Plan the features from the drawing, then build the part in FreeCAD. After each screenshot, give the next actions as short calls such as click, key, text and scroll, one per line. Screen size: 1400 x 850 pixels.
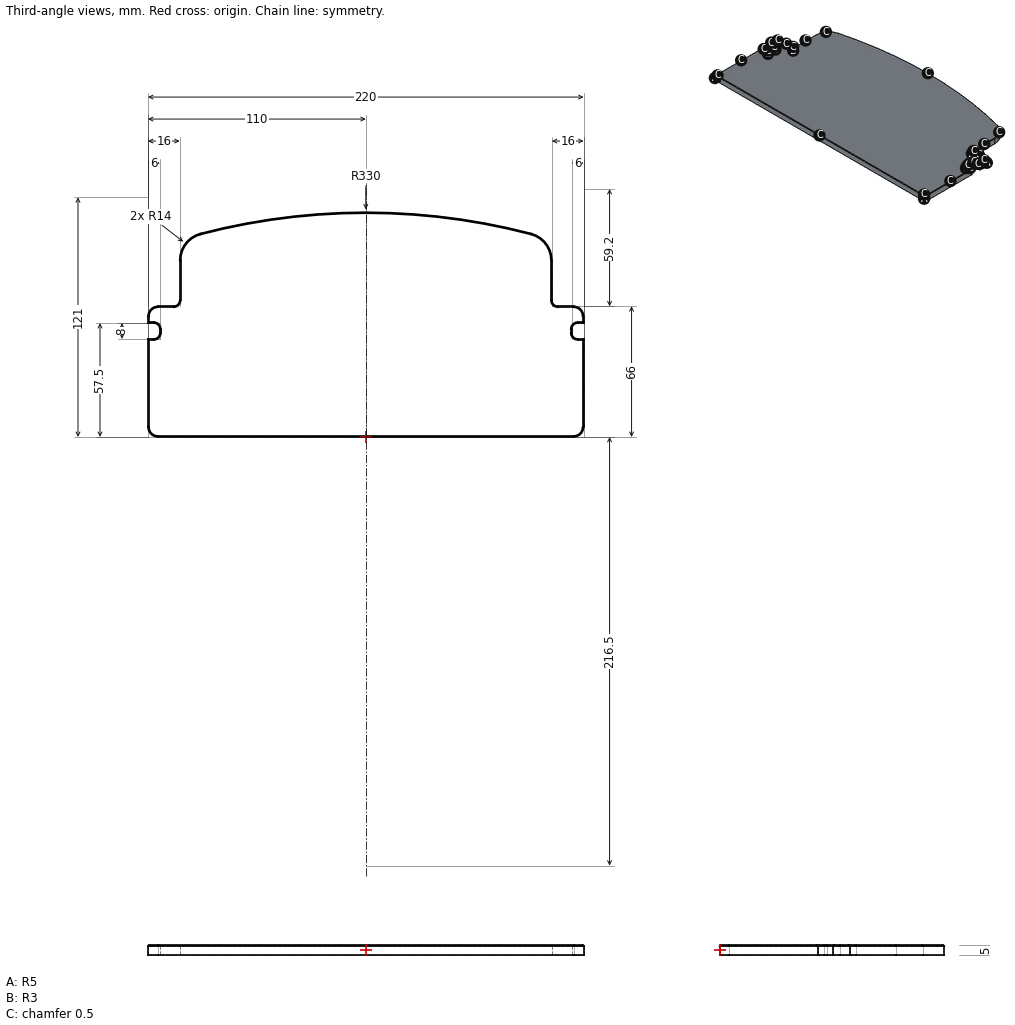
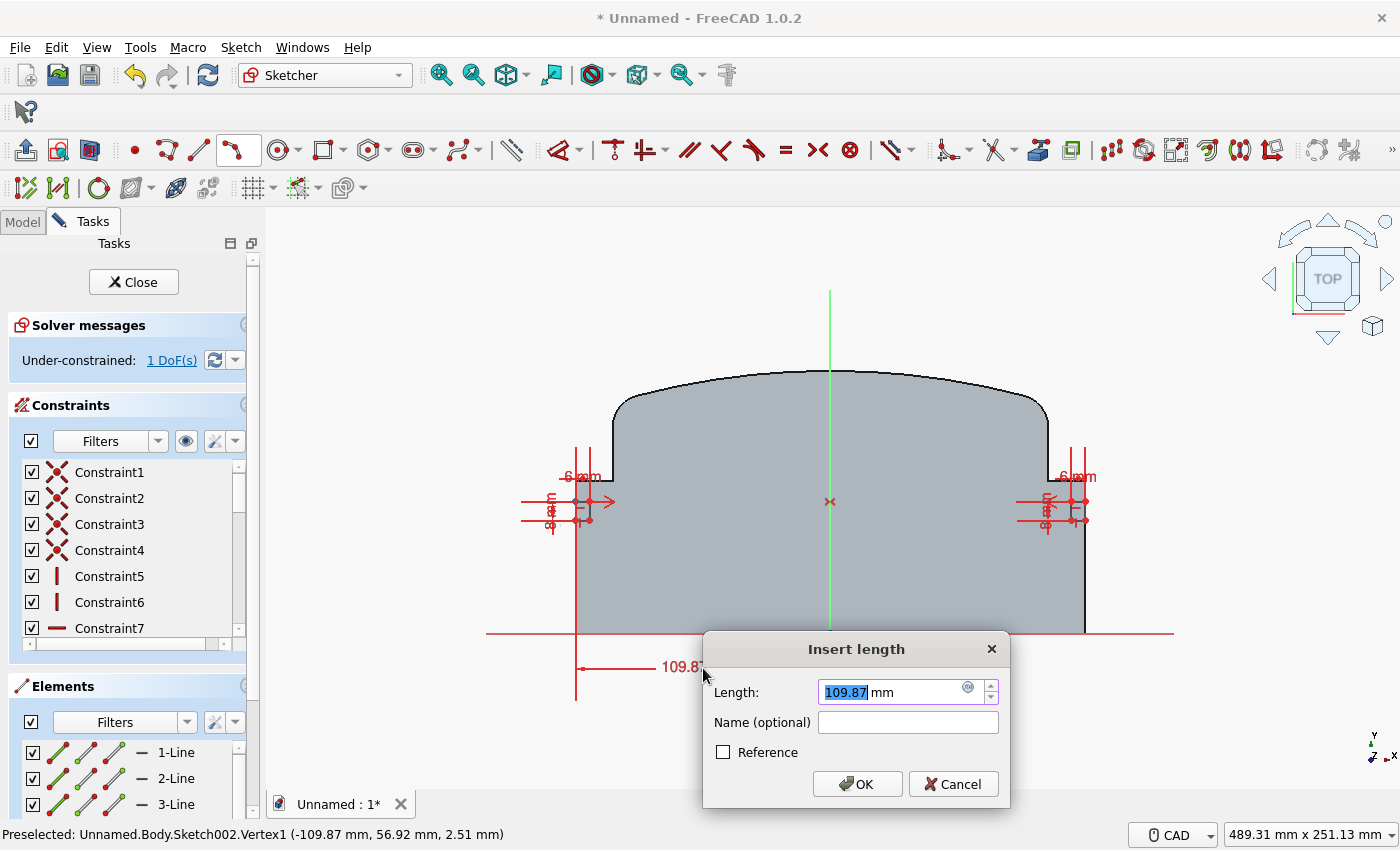
text(110)
key(Return)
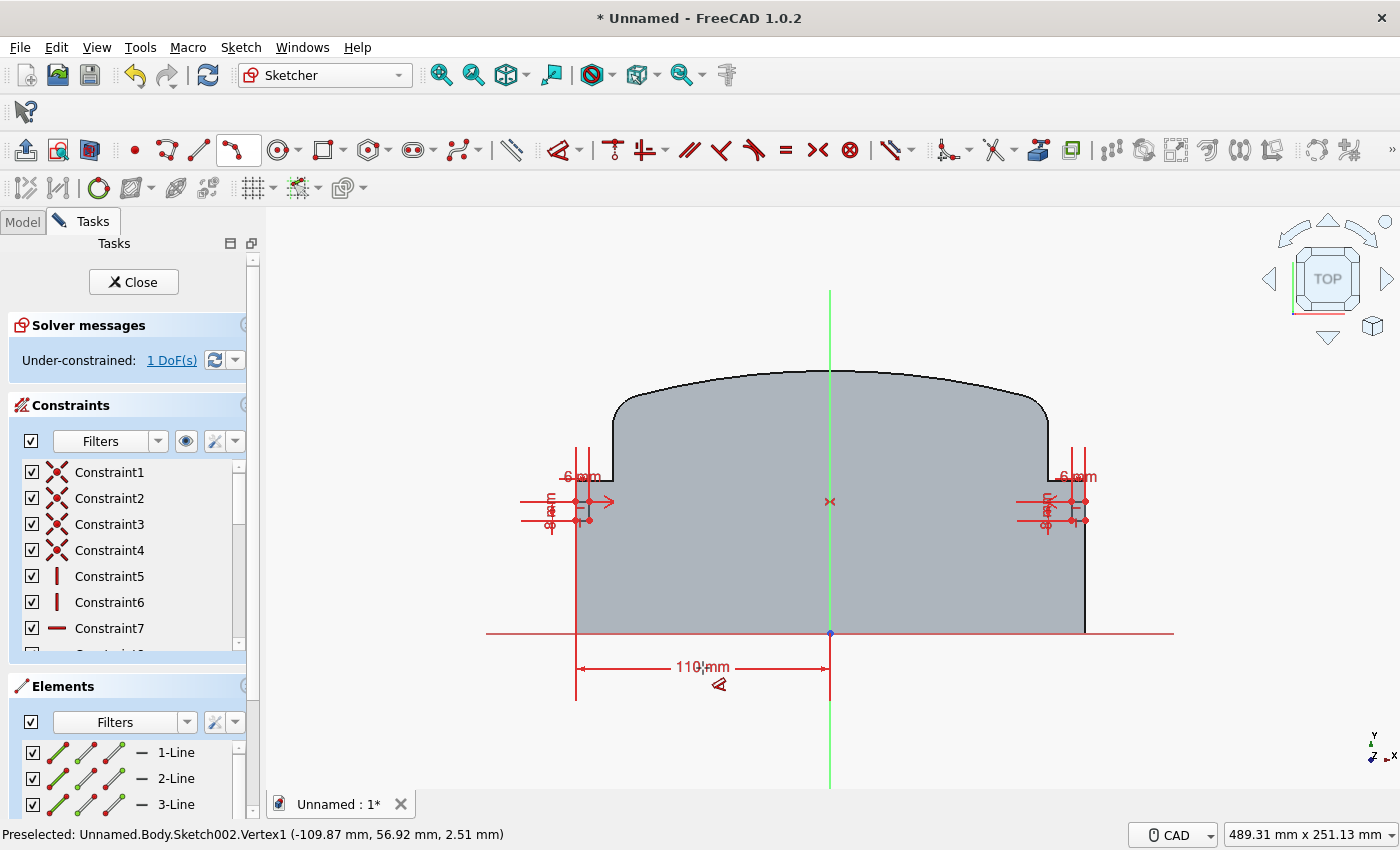
click(576, 502)
click(542, 568)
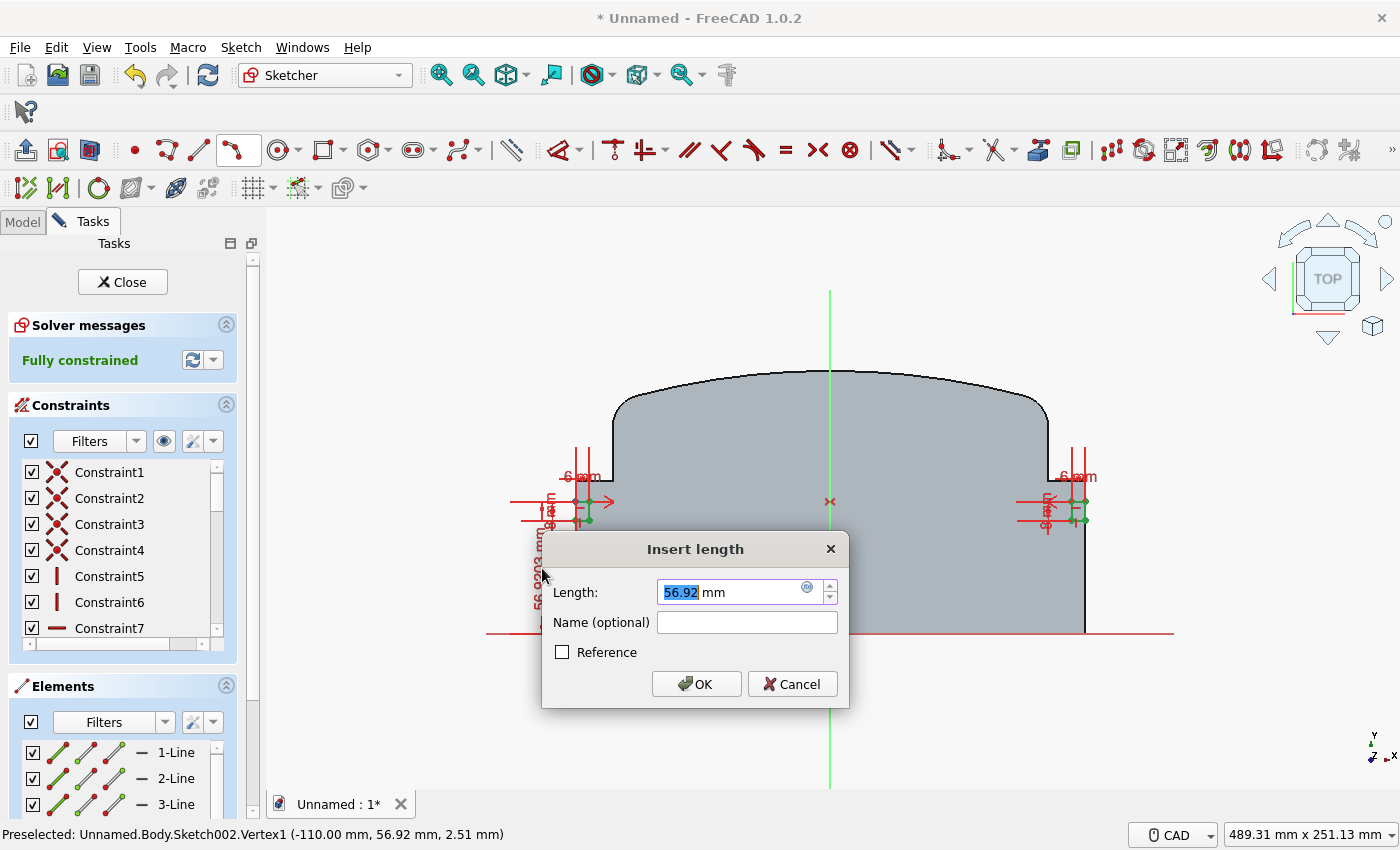
text(57.5)
key(Return)
key(Escape)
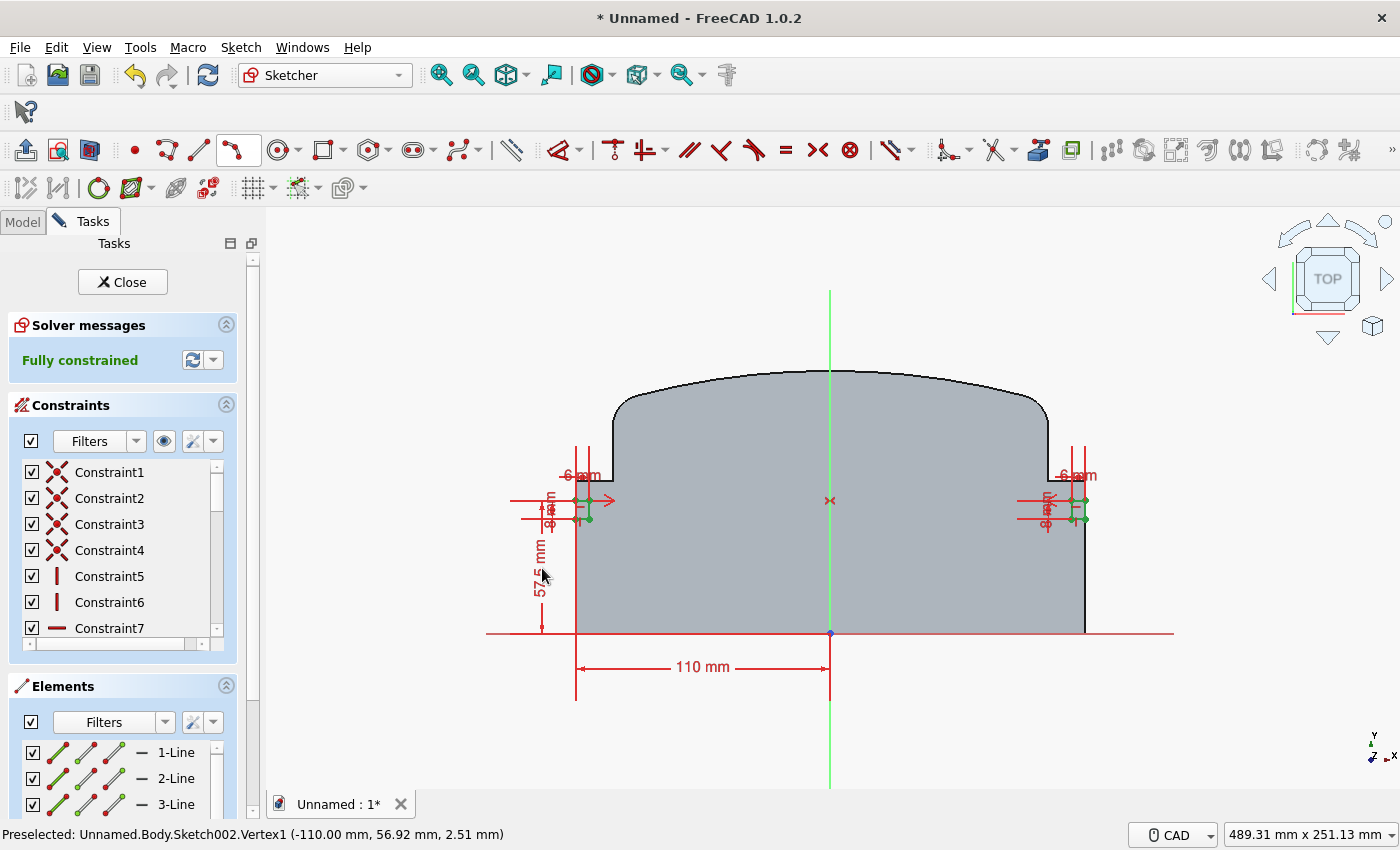
click(123, 282)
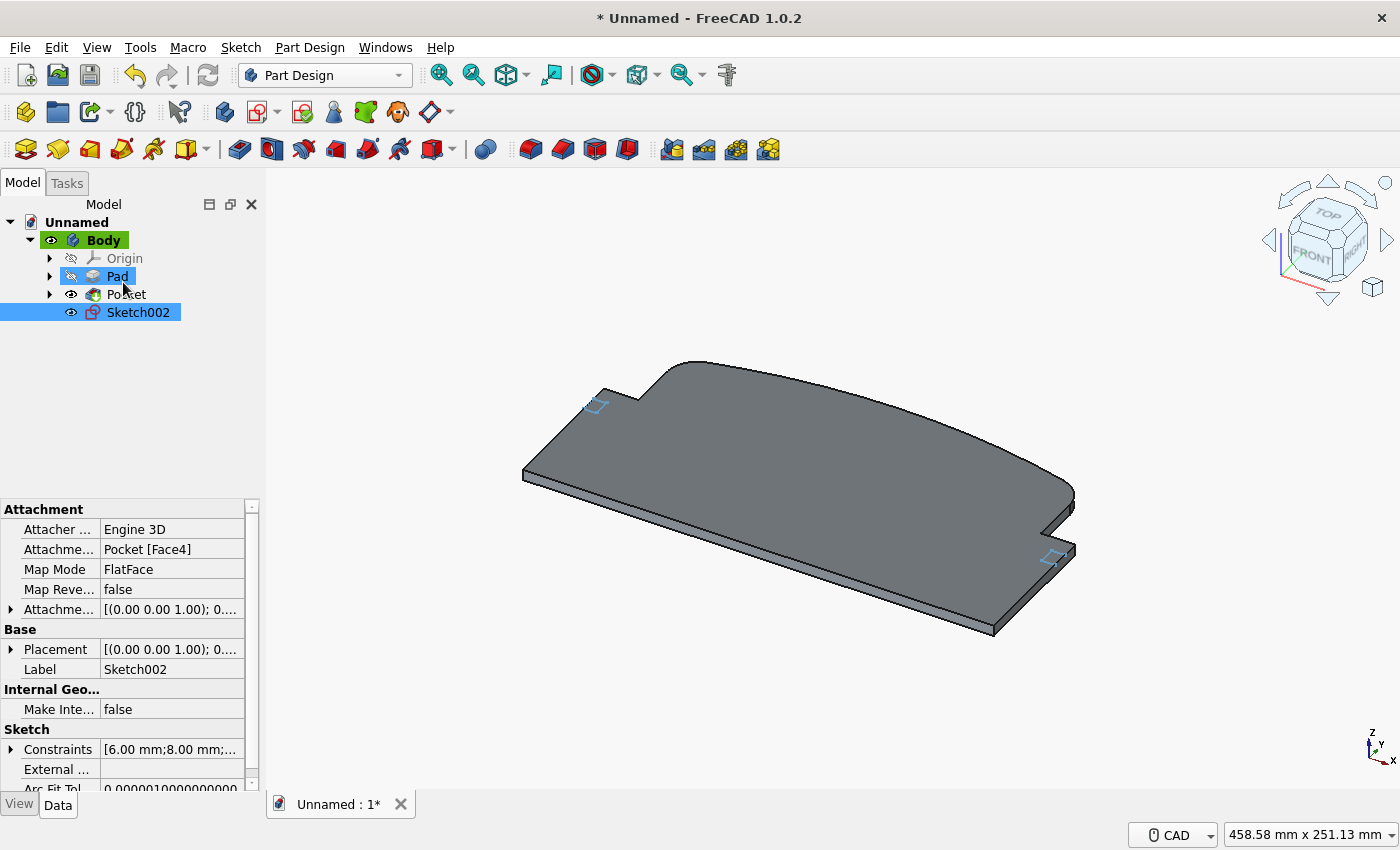
click(240, 150)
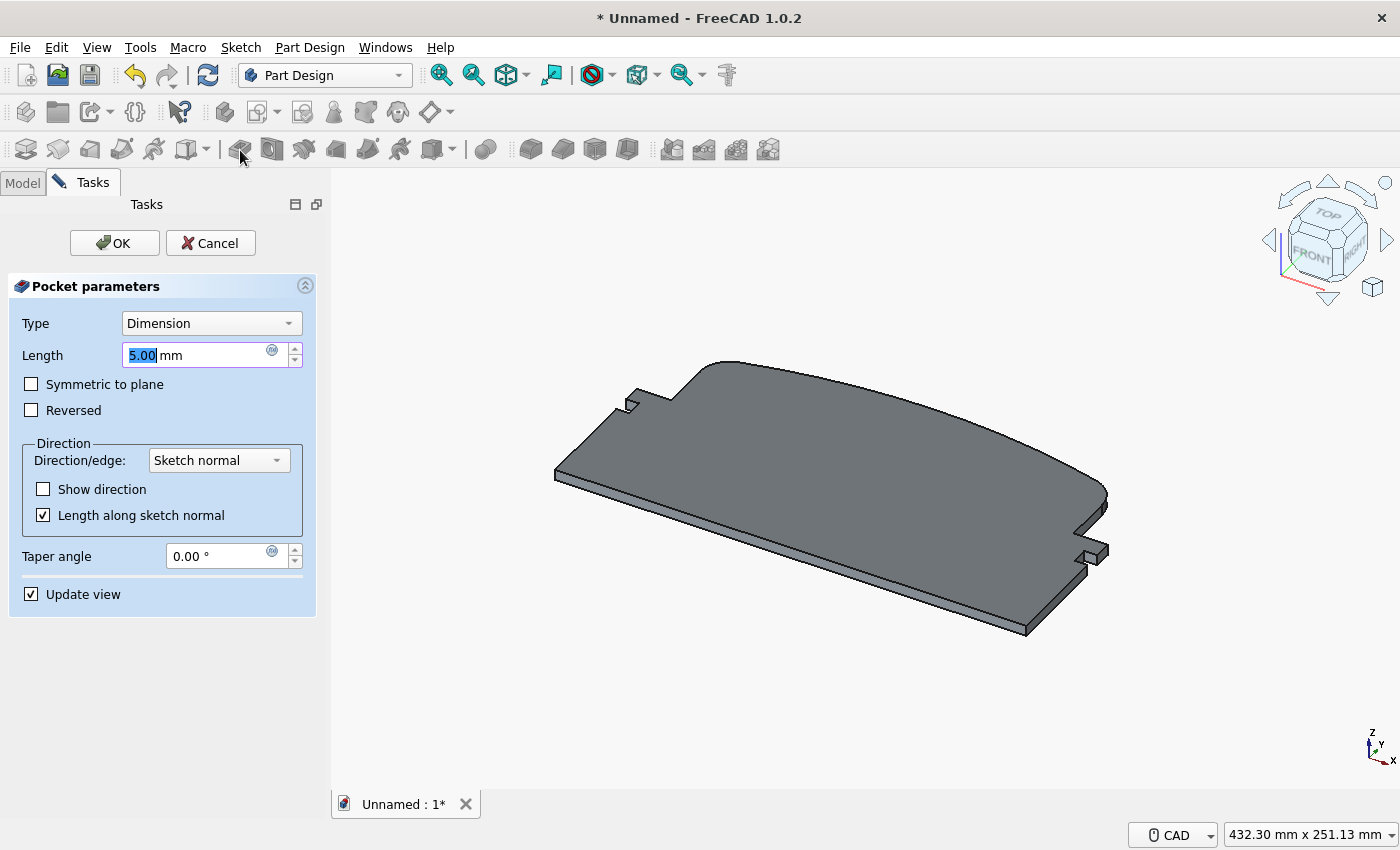
click(212, 324)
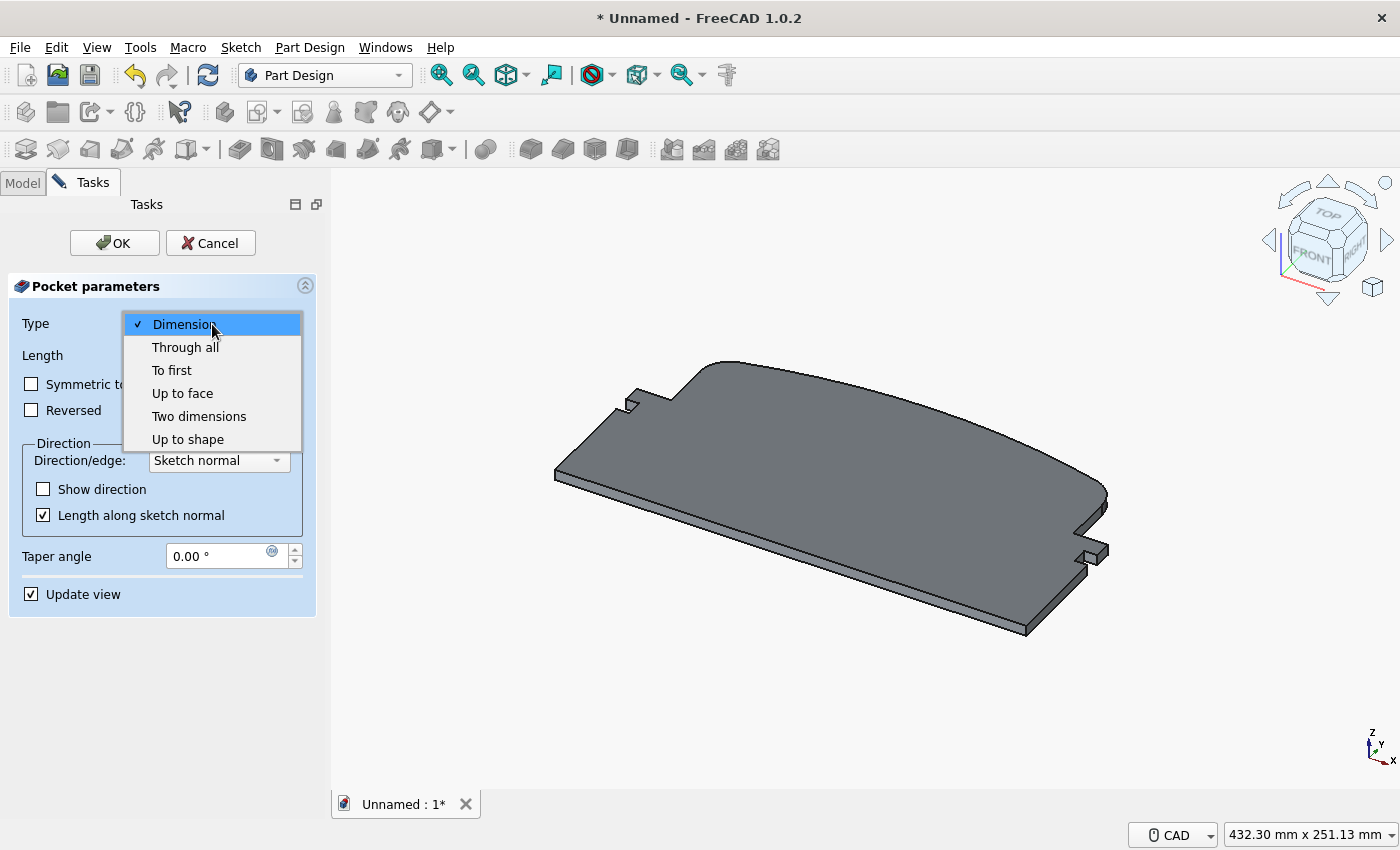
click(212, 348)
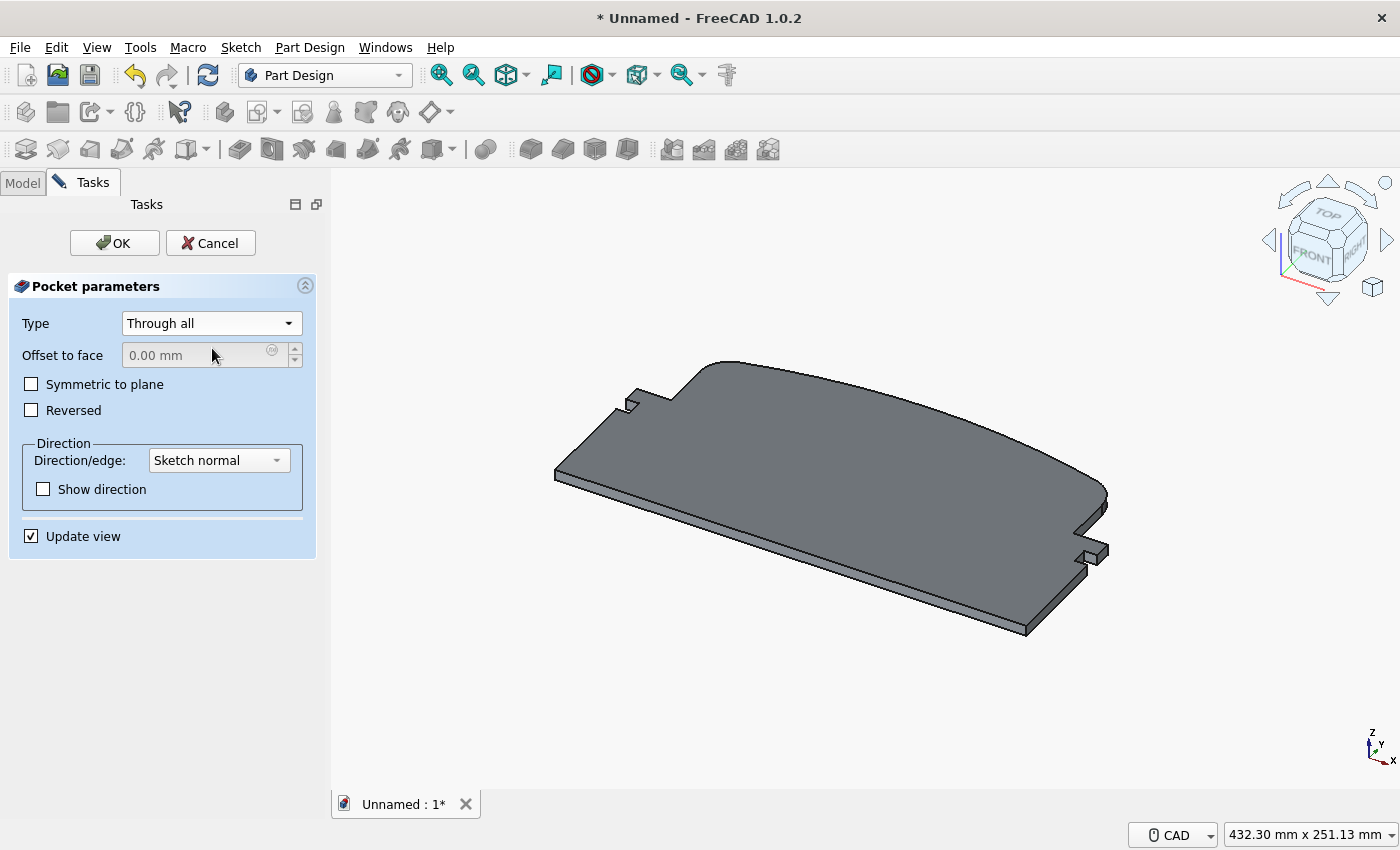
click(115, 243)